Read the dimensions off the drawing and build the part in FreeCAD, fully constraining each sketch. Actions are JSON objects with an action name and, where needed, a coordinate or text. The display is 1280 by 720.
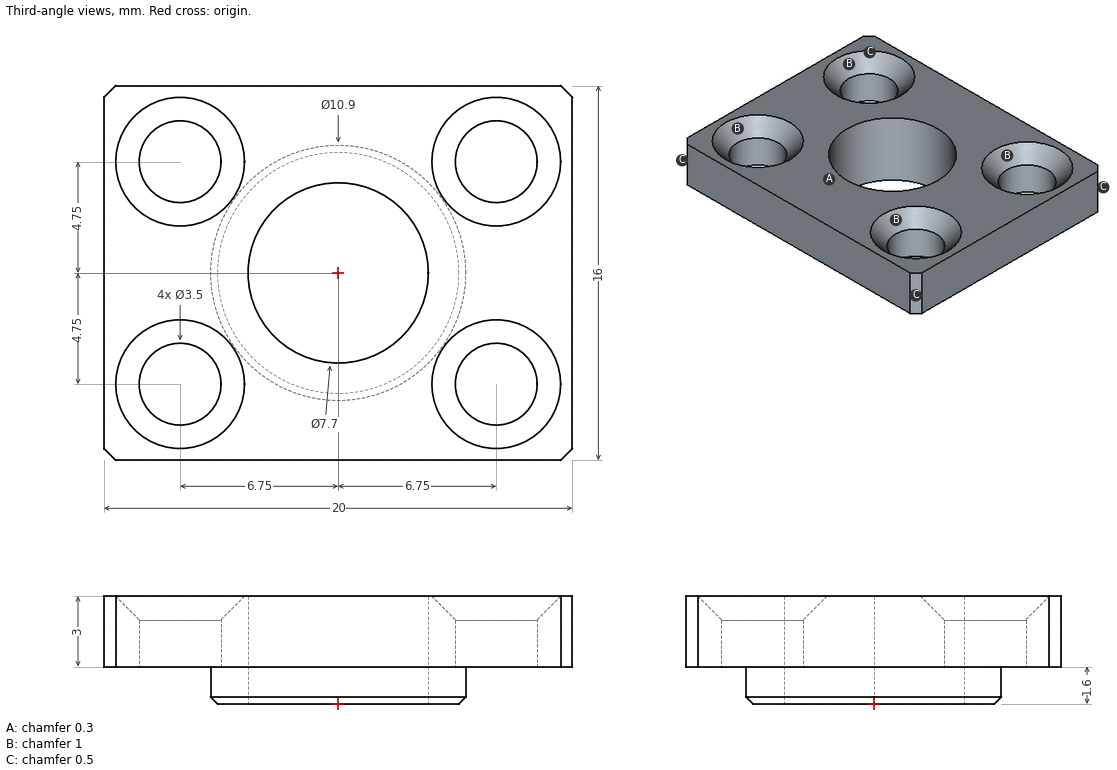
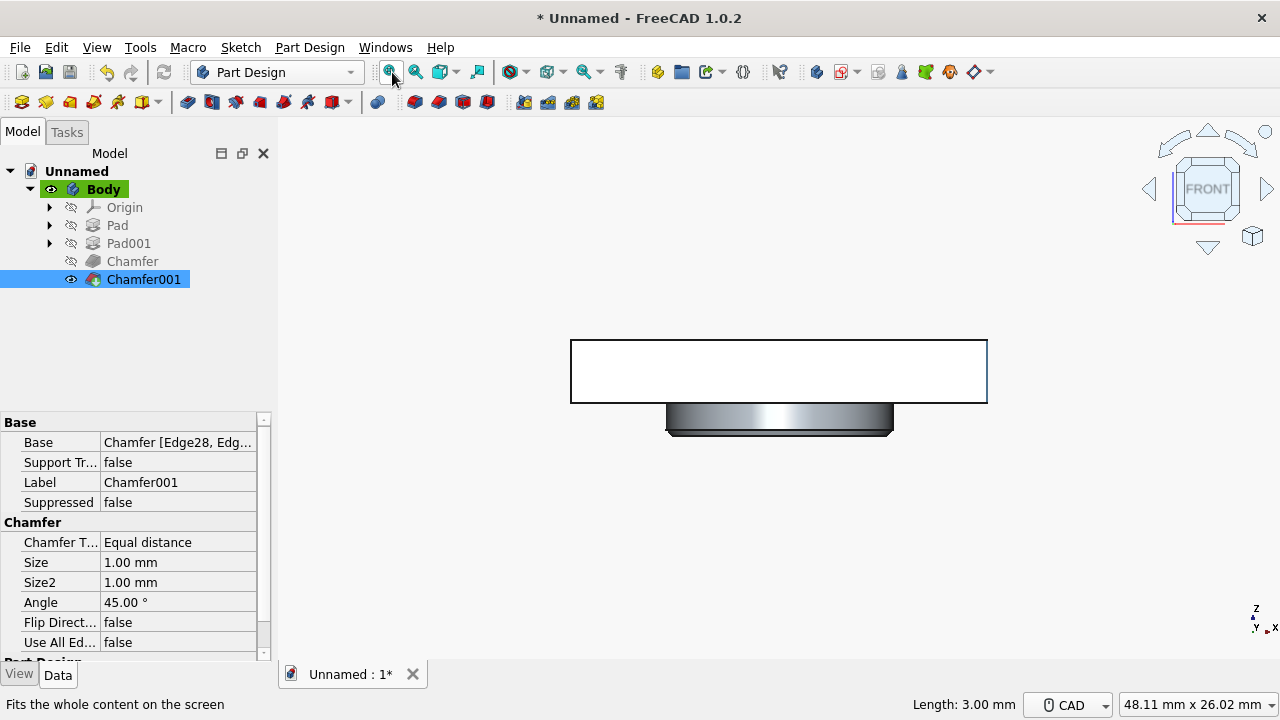
{"action": "left_click", "coordinate": [571, 370], "text": "ctrl"}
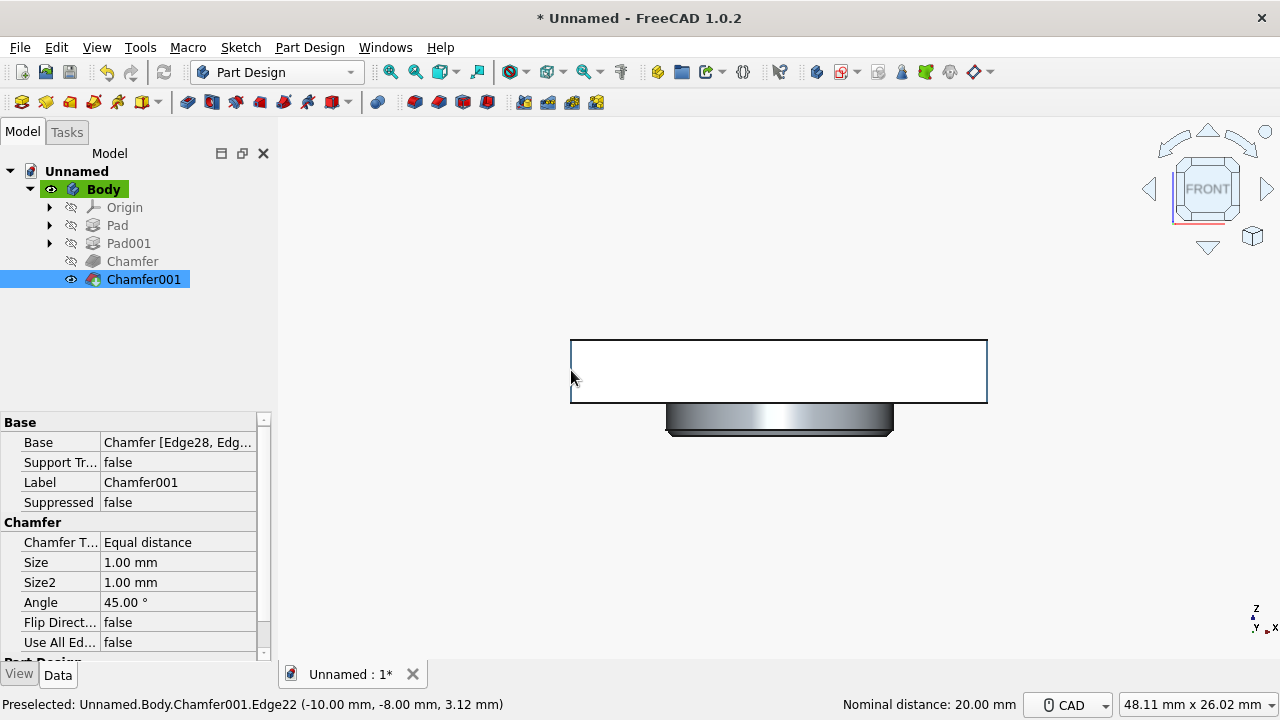
{"action": "key", "text": "3"}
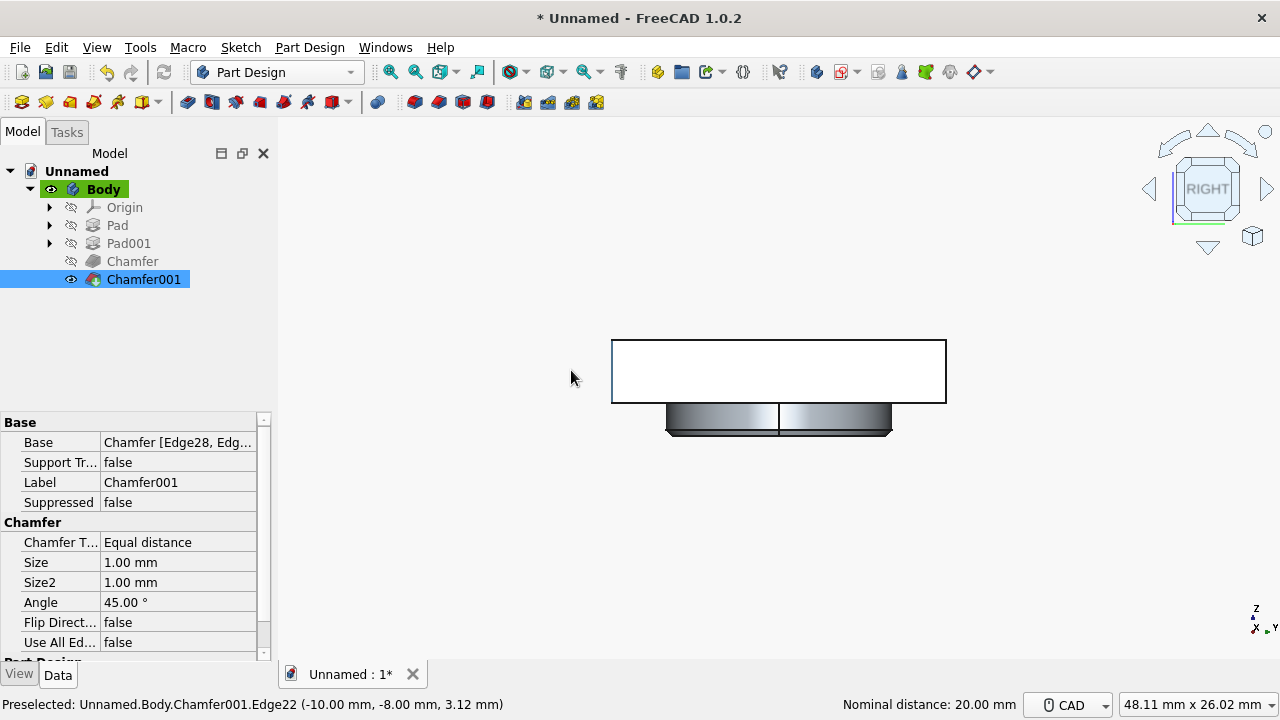
{"action": "key", "text": "v f"}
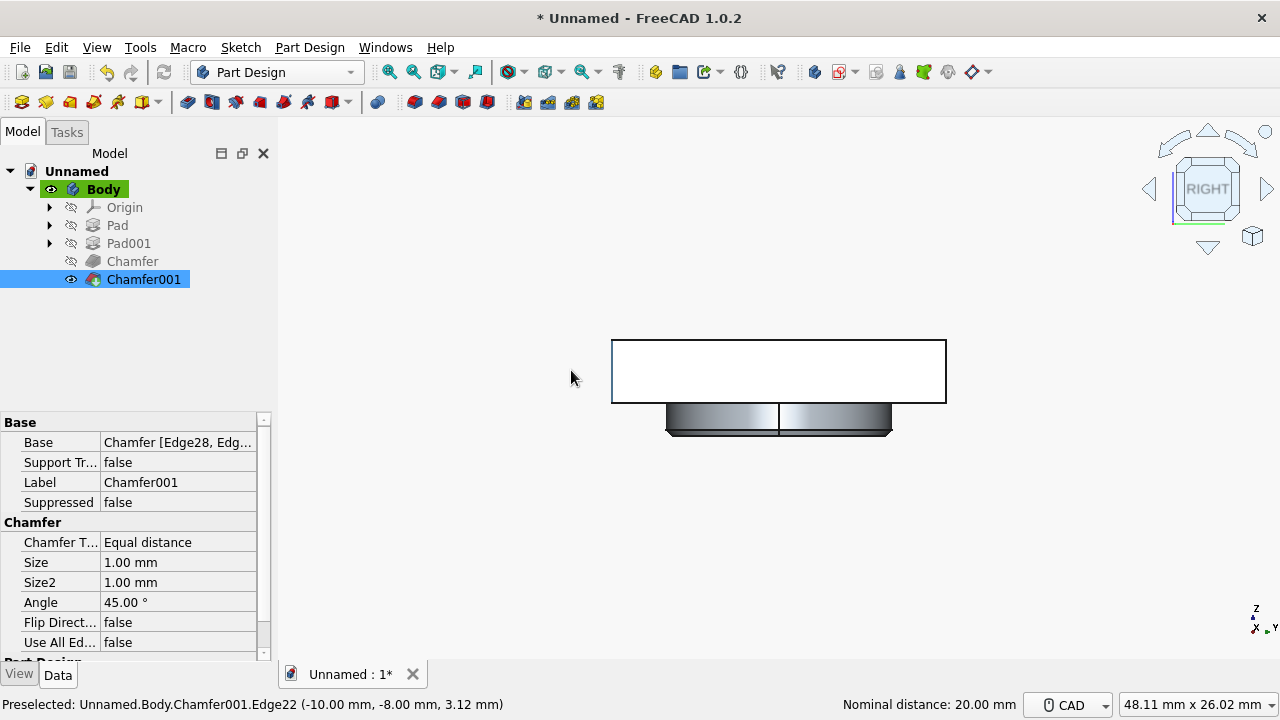
{"action": "left_click", "coordinate": [946, 370], "text": "ctrl"}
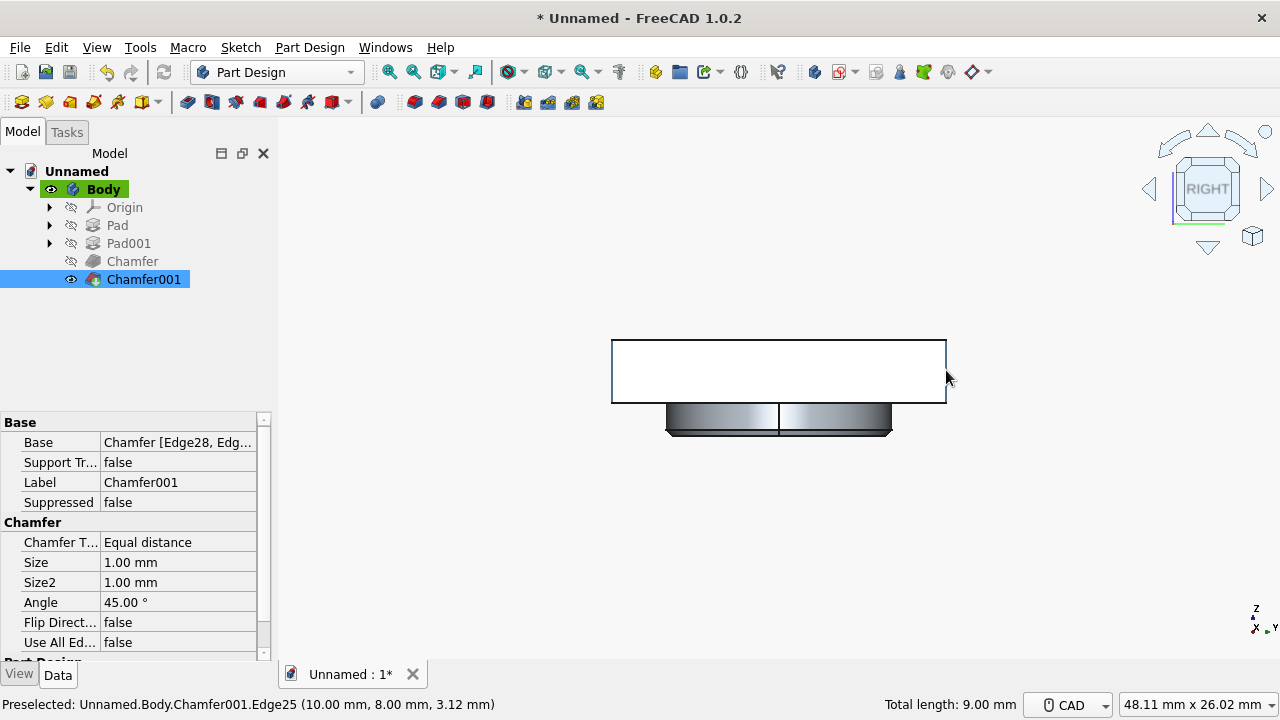
{"action": "key", "text": "5"}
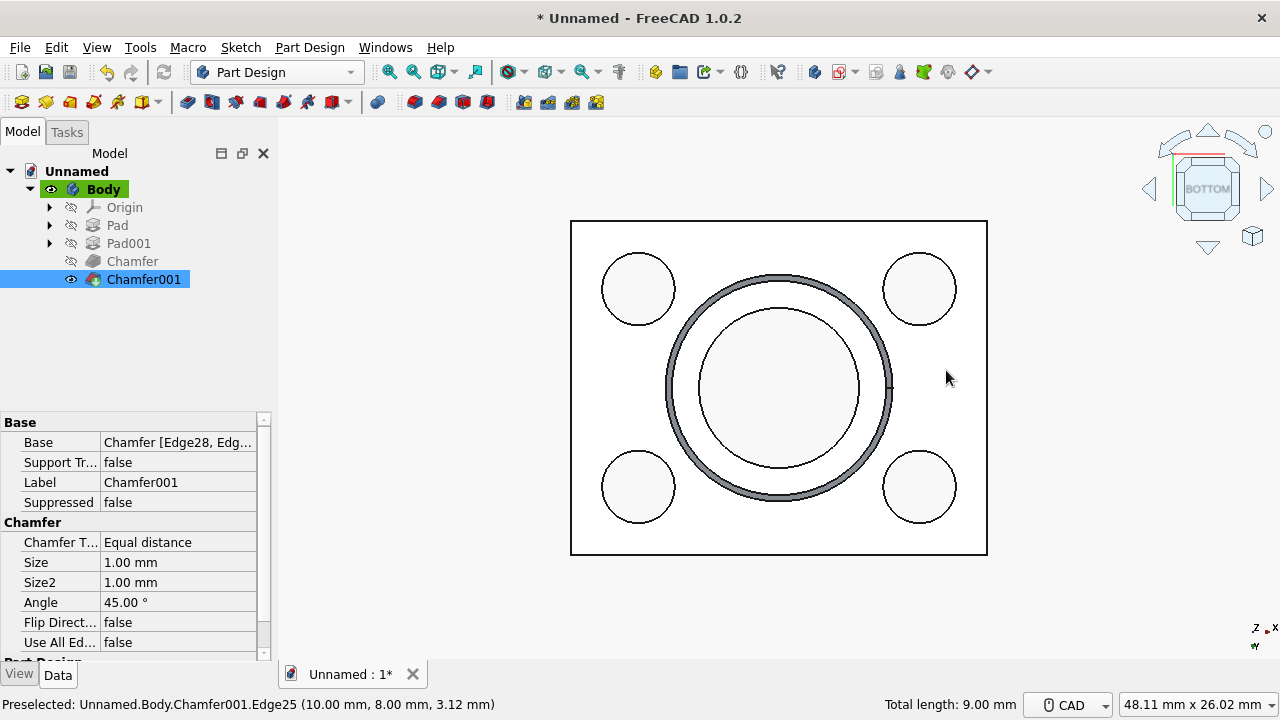
{"action": "key", "text": "4"}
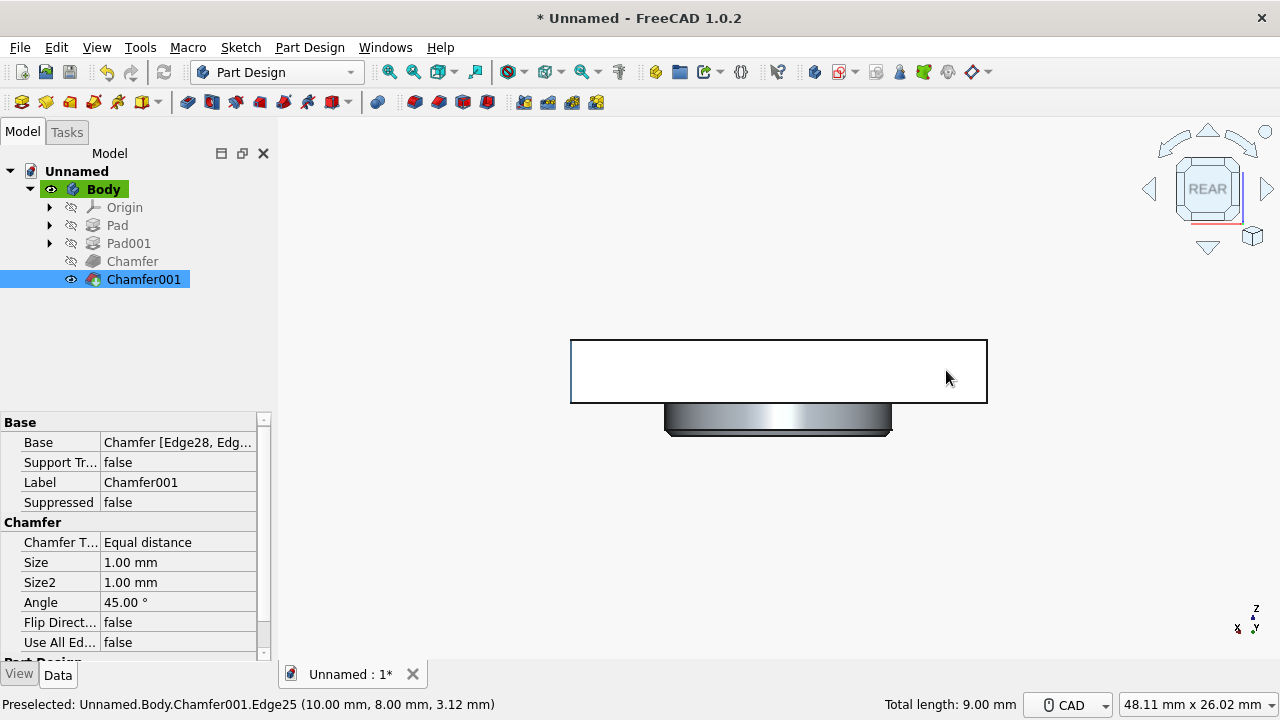
{"action": "left_click", "coordinate": [390, 72]}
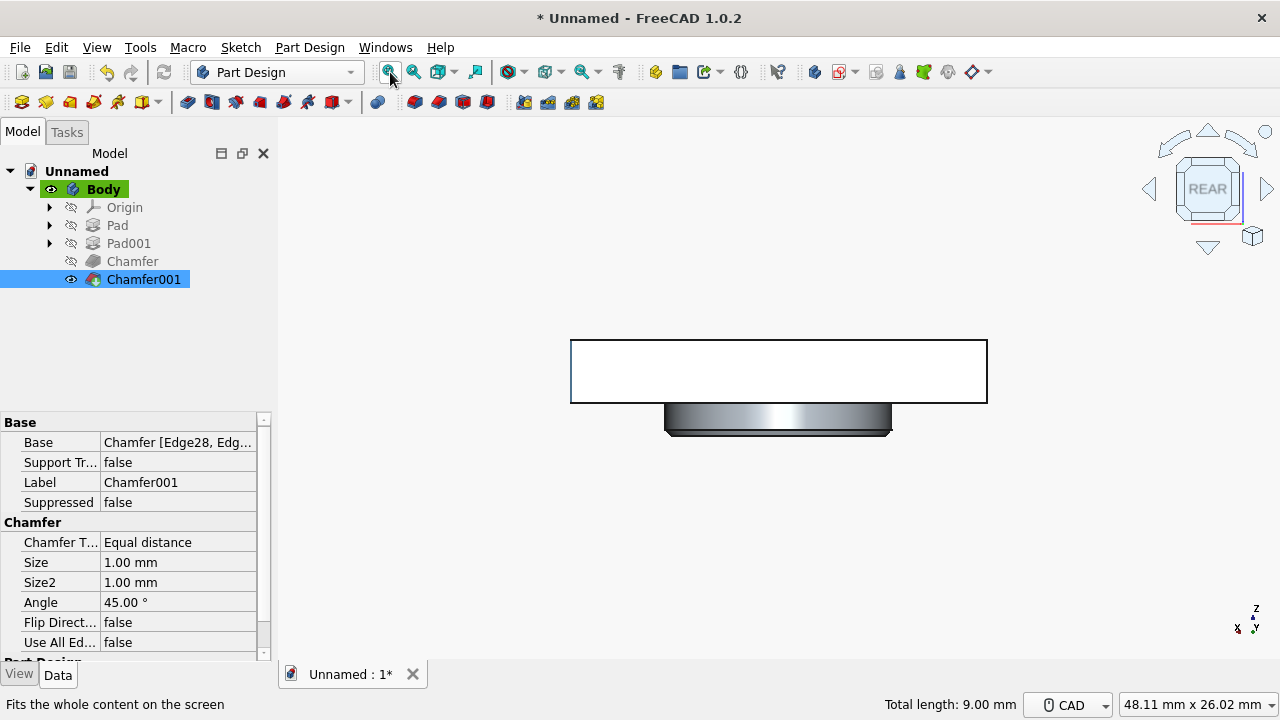
{"action": "left_click", "coordinate": [987, 370], "text": "ctrl"}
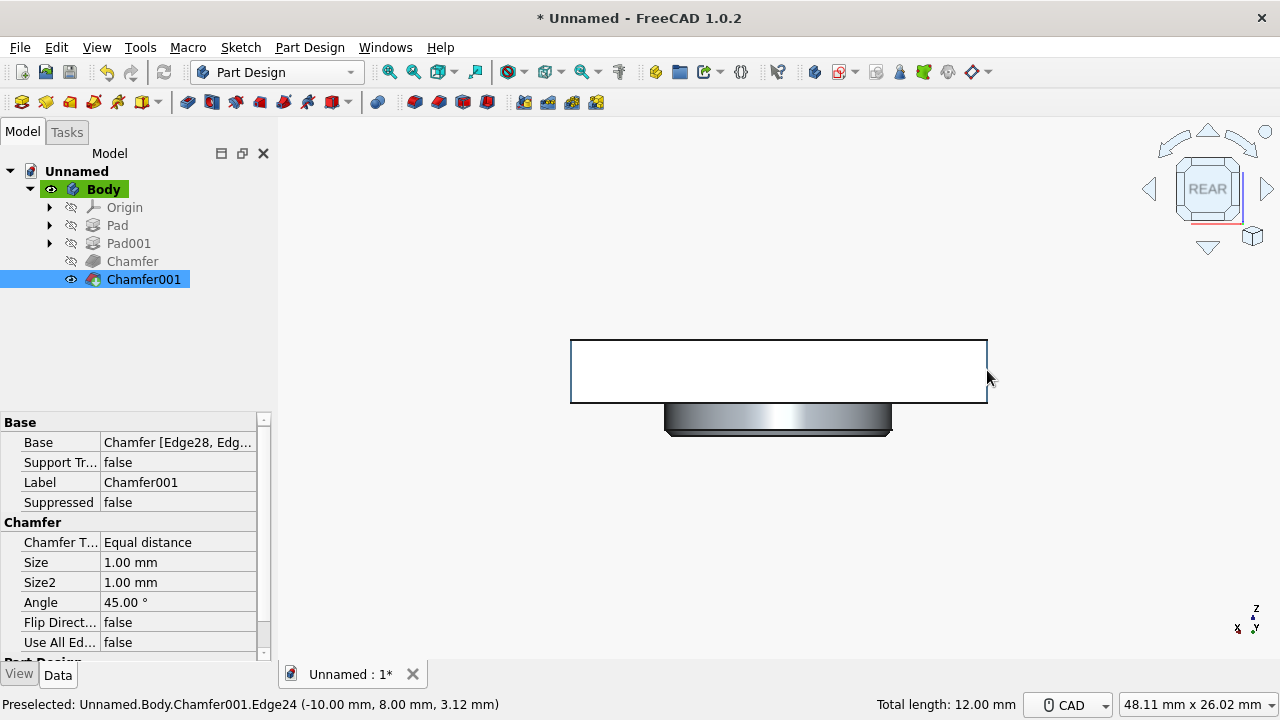
{"action": "left_click", "coordinate": [440, 102]}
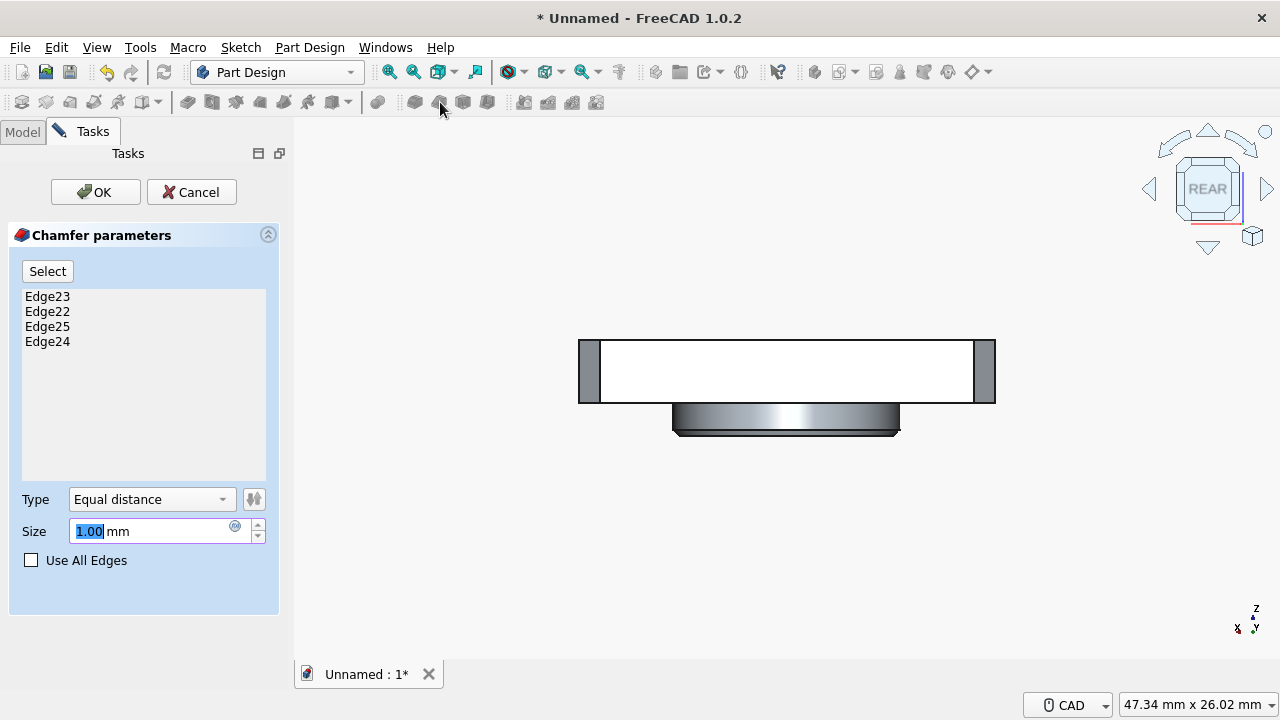
{"action": "type", "text": "0.5"}
{"action": "key", "text": "Tab"}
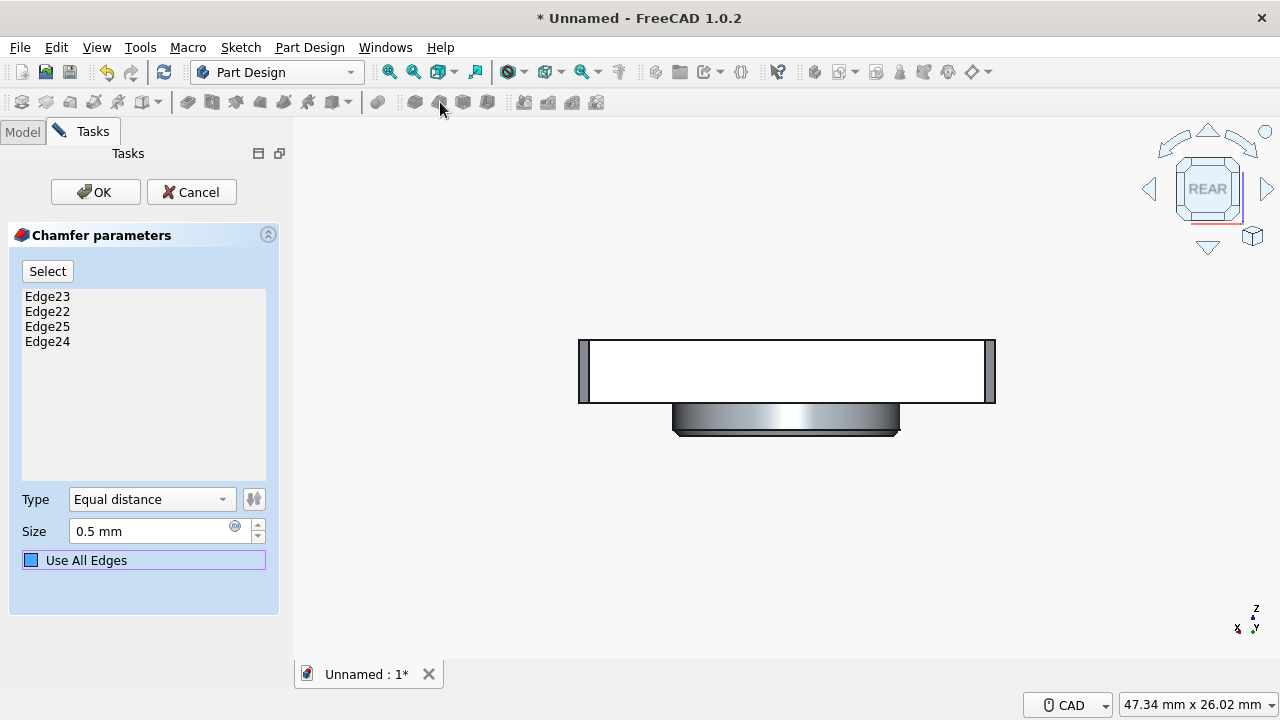
{"action": "left_click", "coordinate": [96, 192]}